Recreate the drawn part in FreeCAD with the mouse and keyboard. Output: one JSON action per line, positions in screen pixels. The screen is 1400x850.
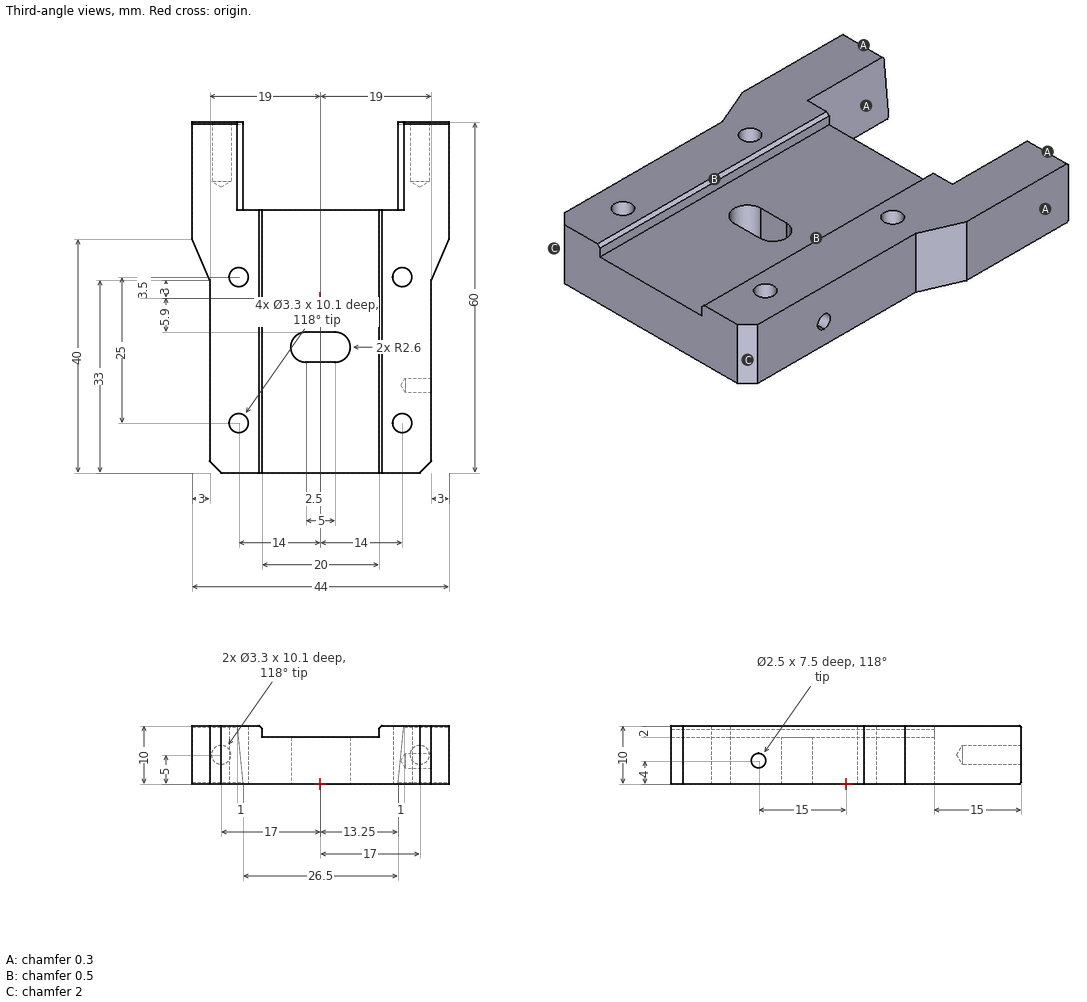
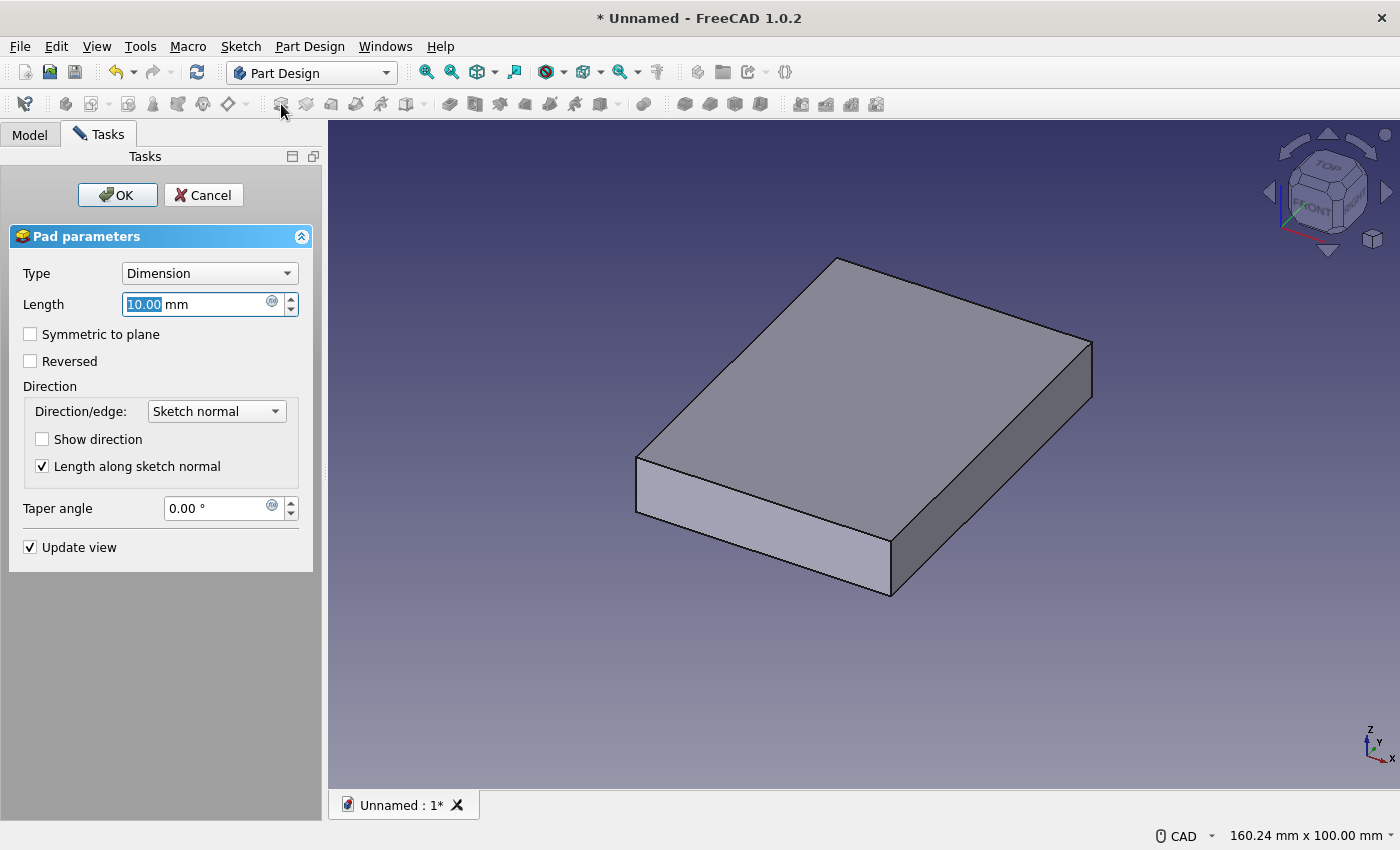
{"action": "type", "text": "10"}
{"action": "key", "text": "Tab"}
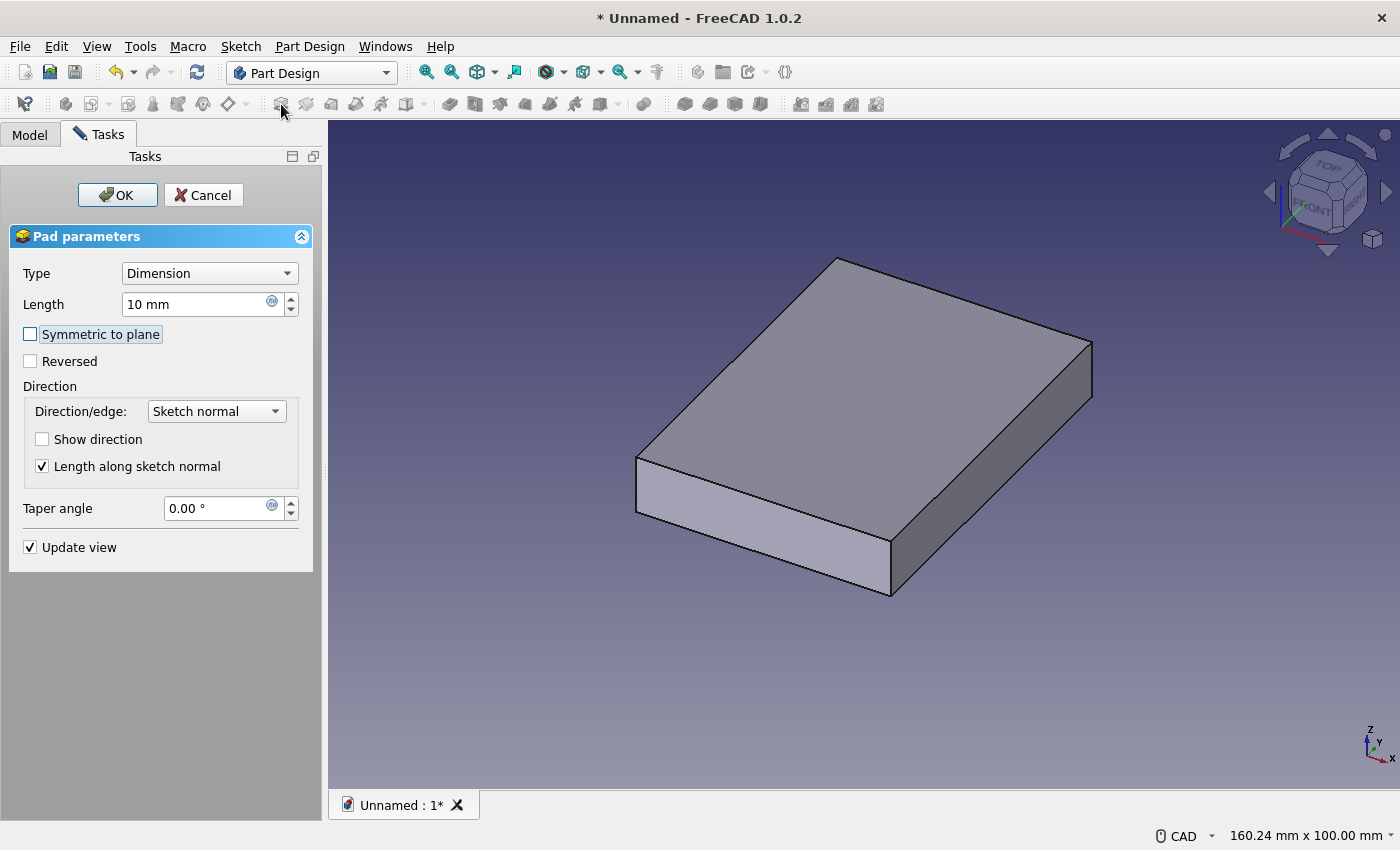
{"action": "left_click", "coordinate": [118, 195]}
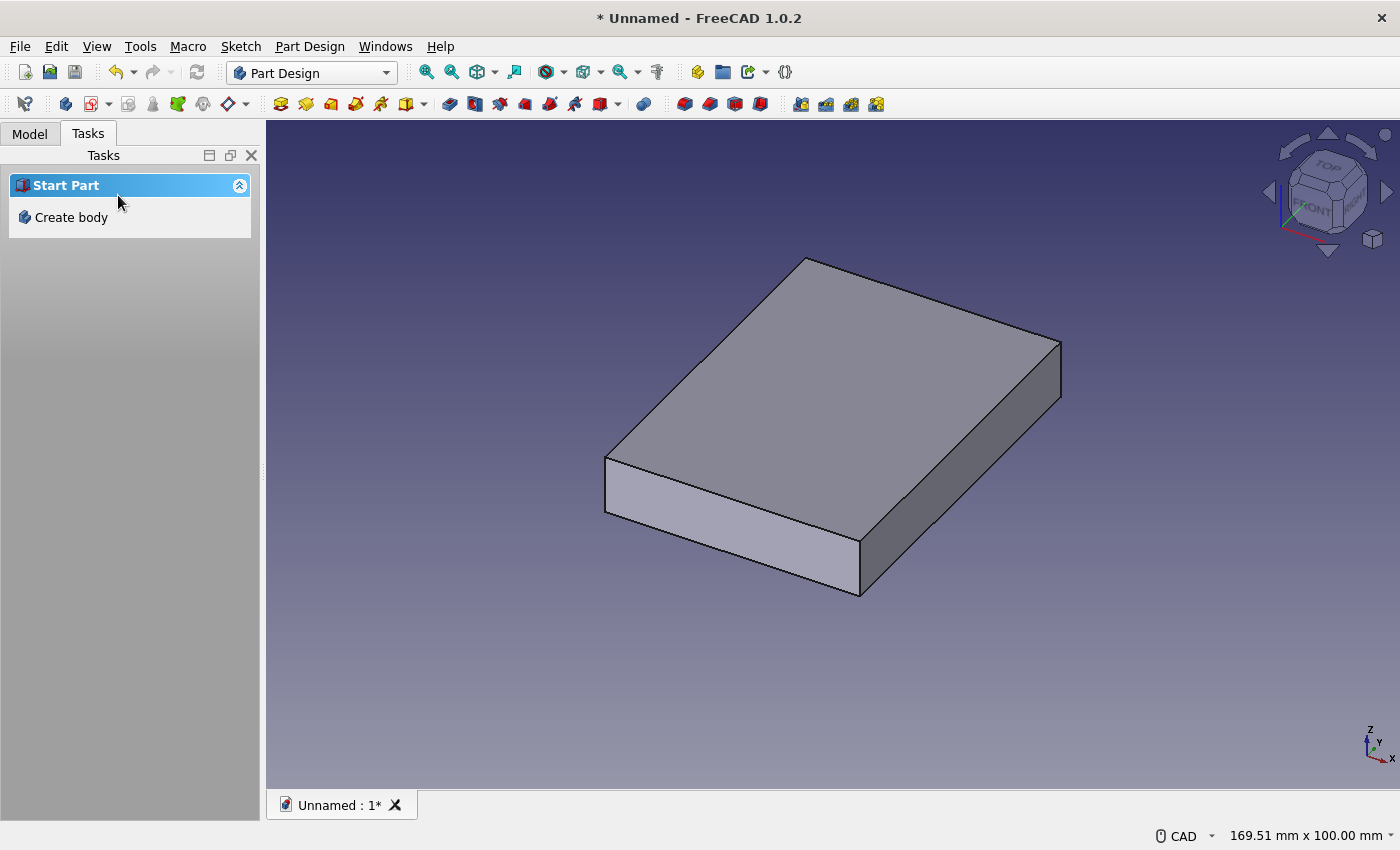
{"action": "key", "text": "4"}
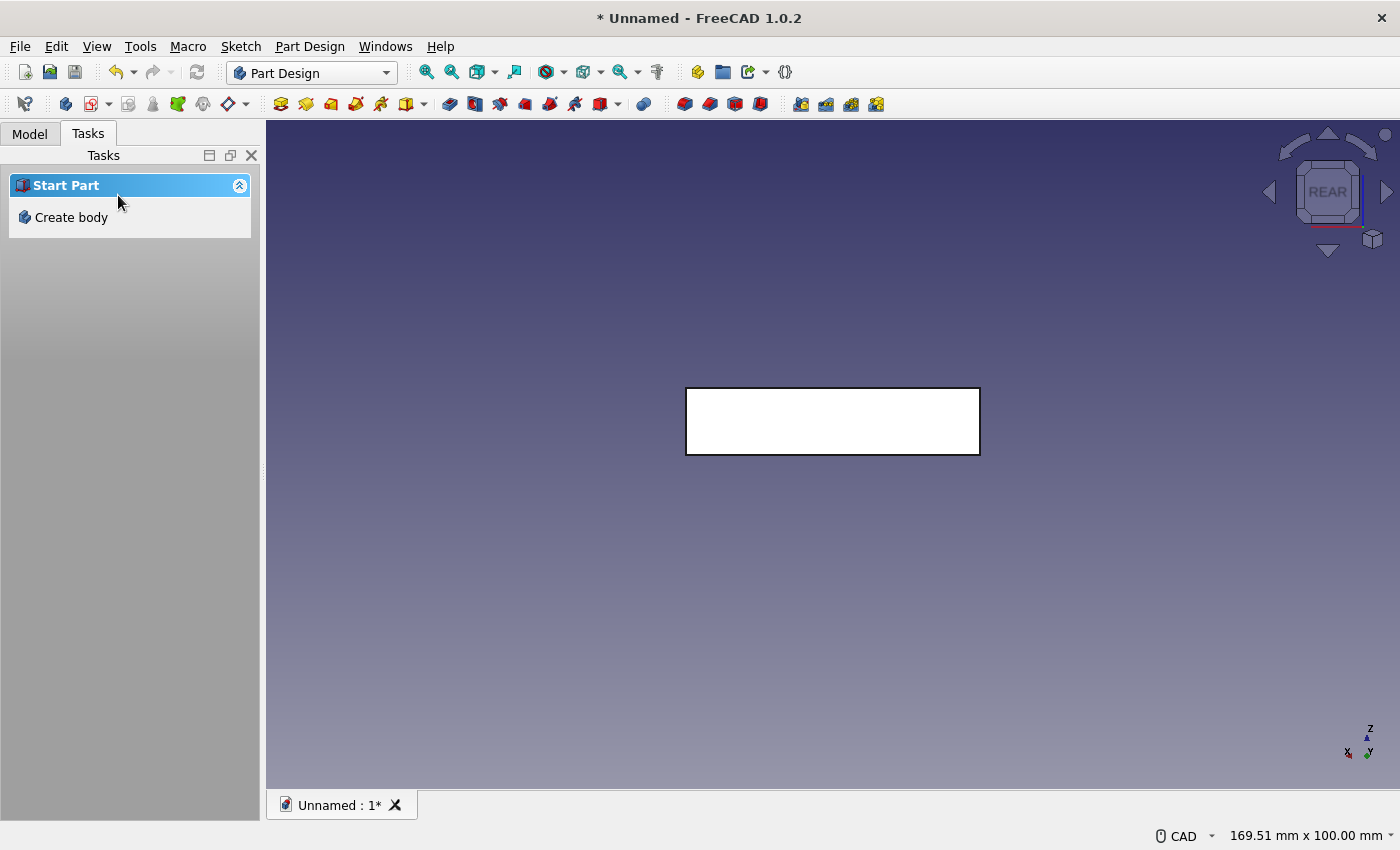
{"action": "left_click", "coordinate": [427, 72]}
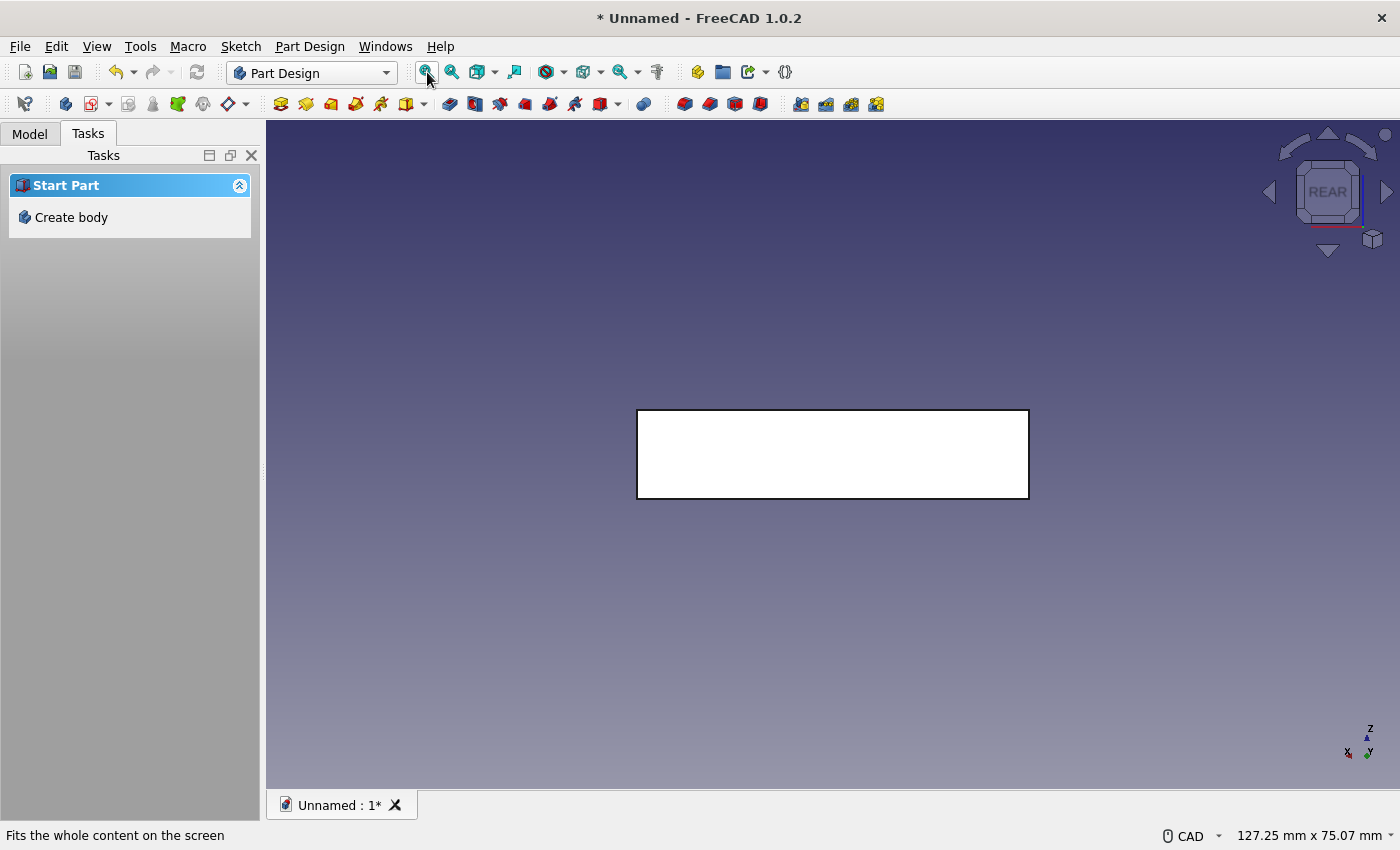
{"action": "left_click", "coordinate": [721, 454]}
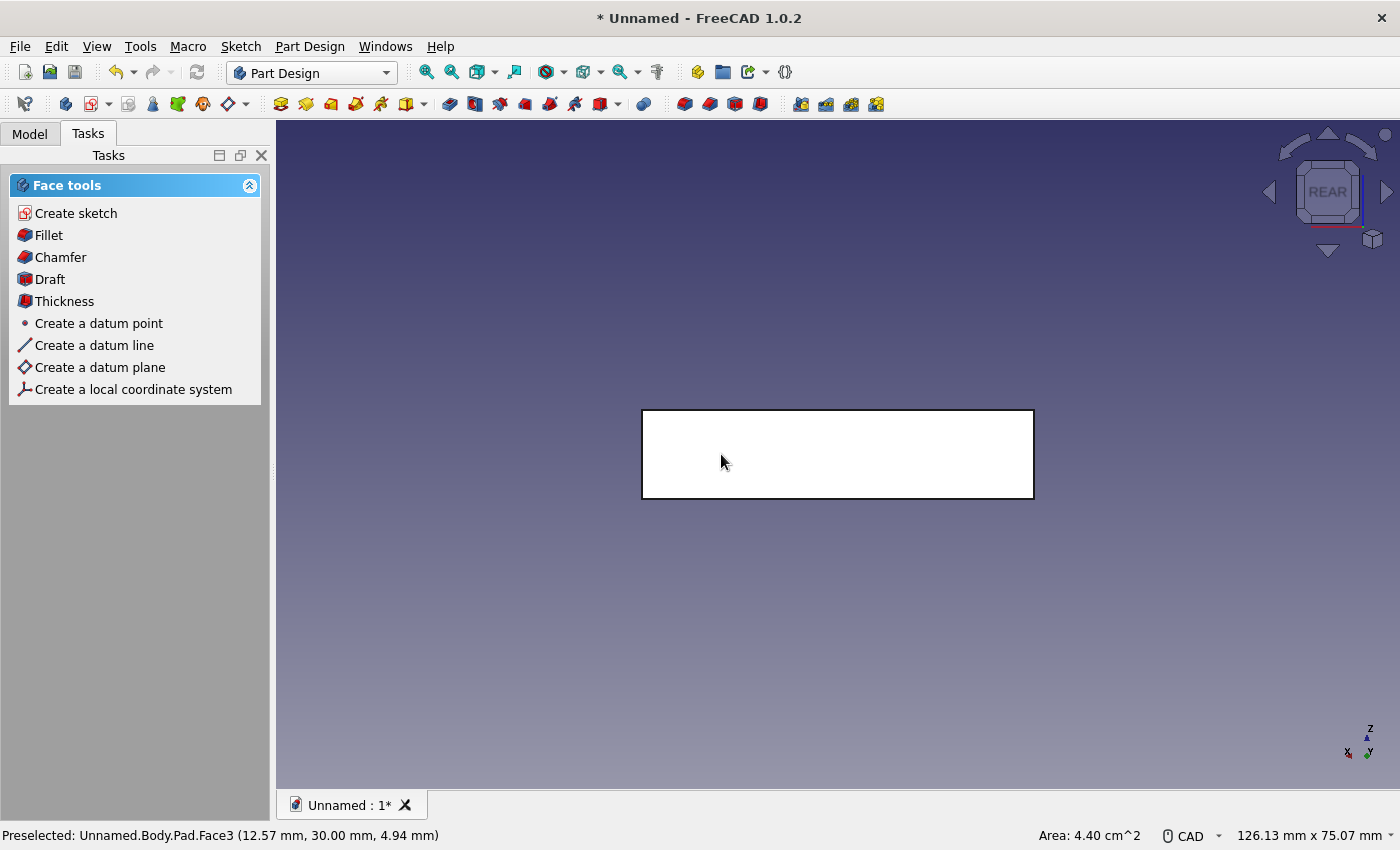
{"action": "left_click", "coordinate": [90, 104]}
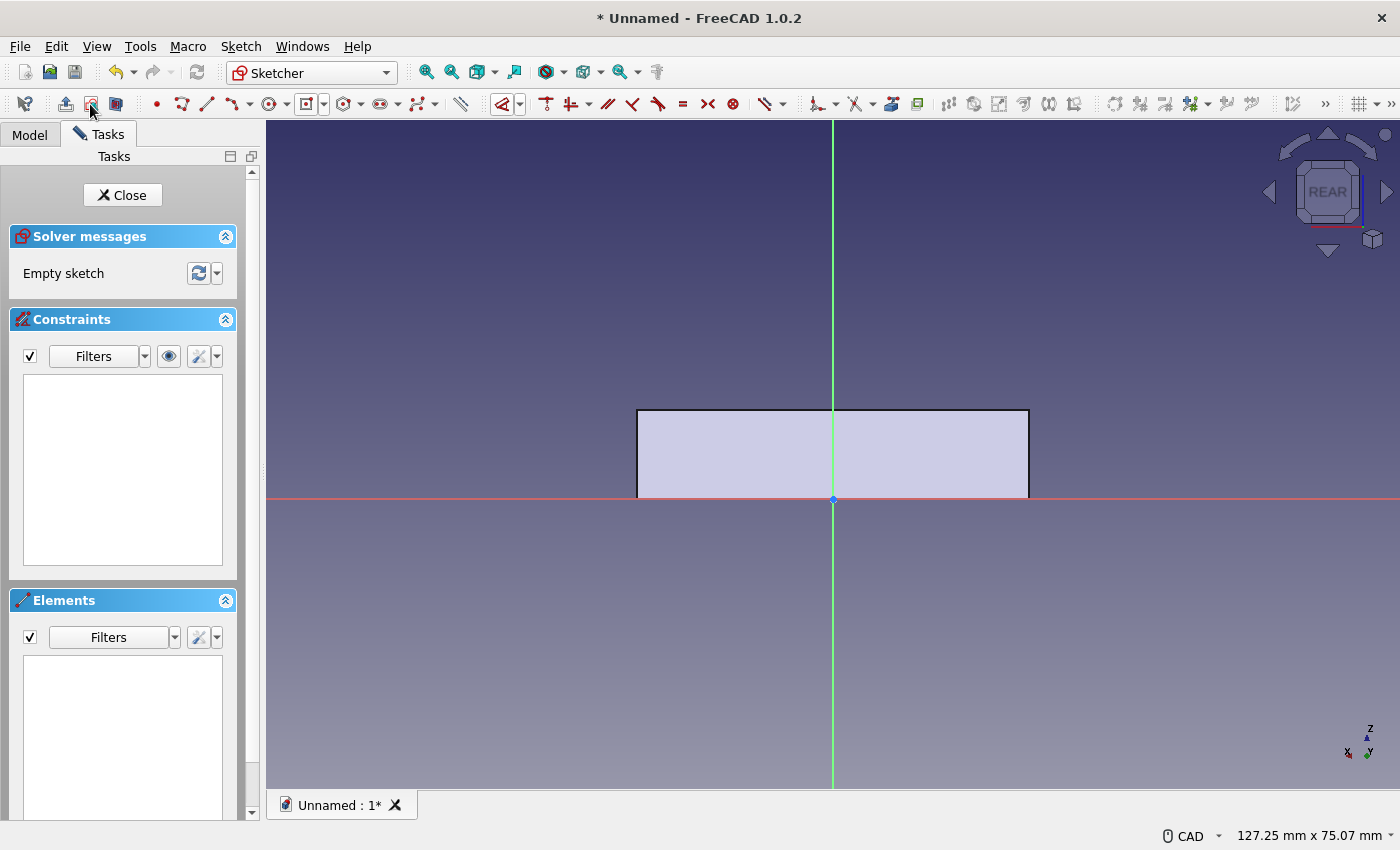
{"action": "scroll", "coordinate": [873, 454], "scroll_direction": "up", "scroll_amount": 5}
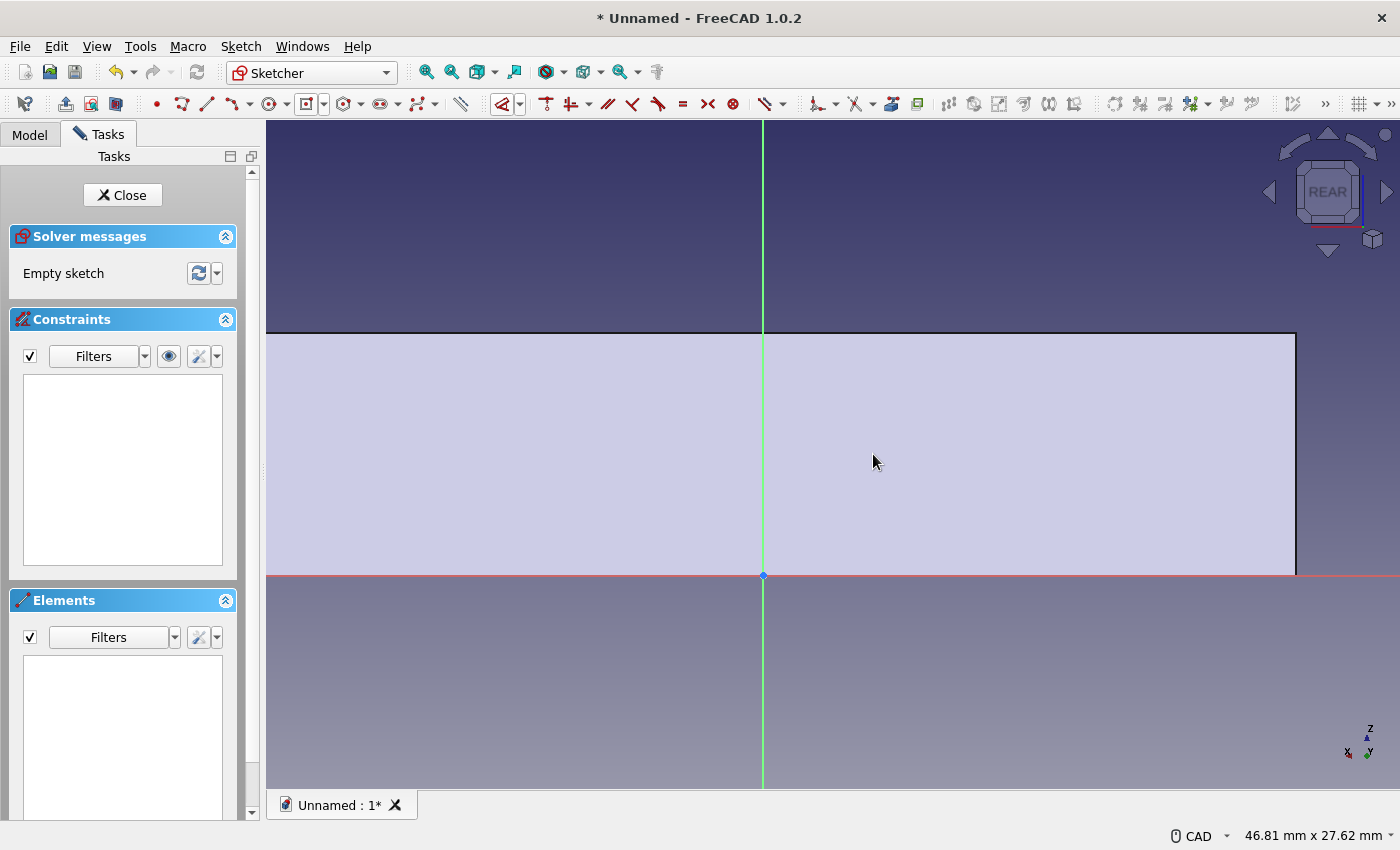
{"action": "left_click", "coordinate": [182, 104]}